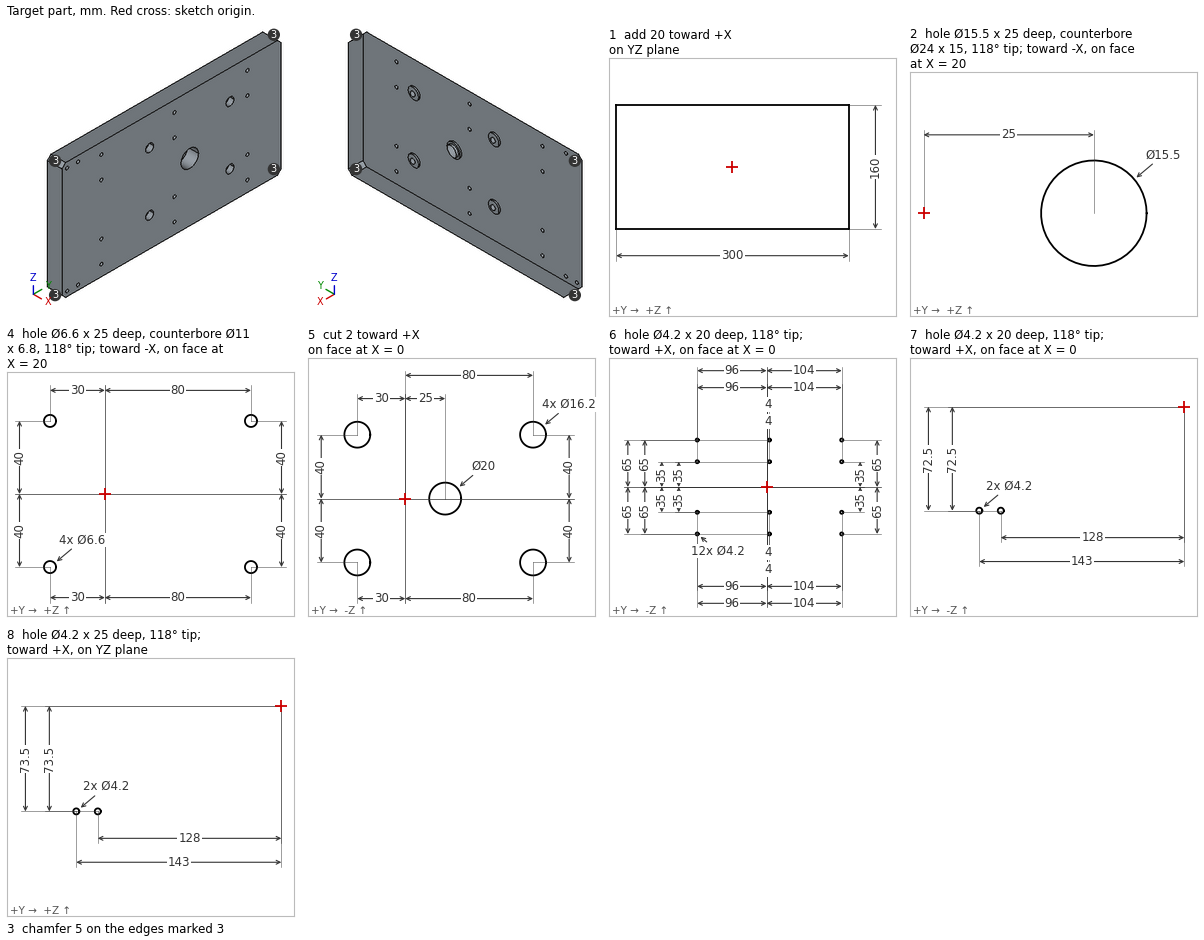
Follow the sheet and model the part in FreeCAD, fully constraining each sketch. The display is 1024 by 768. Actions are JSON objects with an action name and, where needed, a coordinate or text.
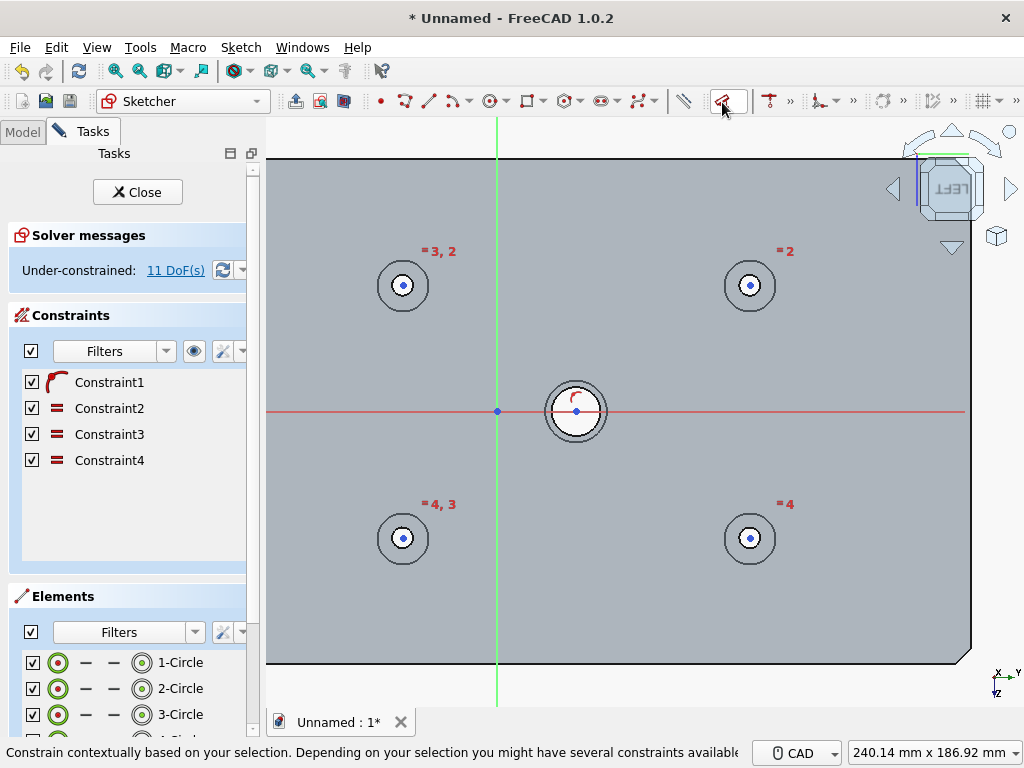
{"action": "left_click", "coordinate": [768, 268]}
{"action": "left_click", "coordinate": [791, 245]}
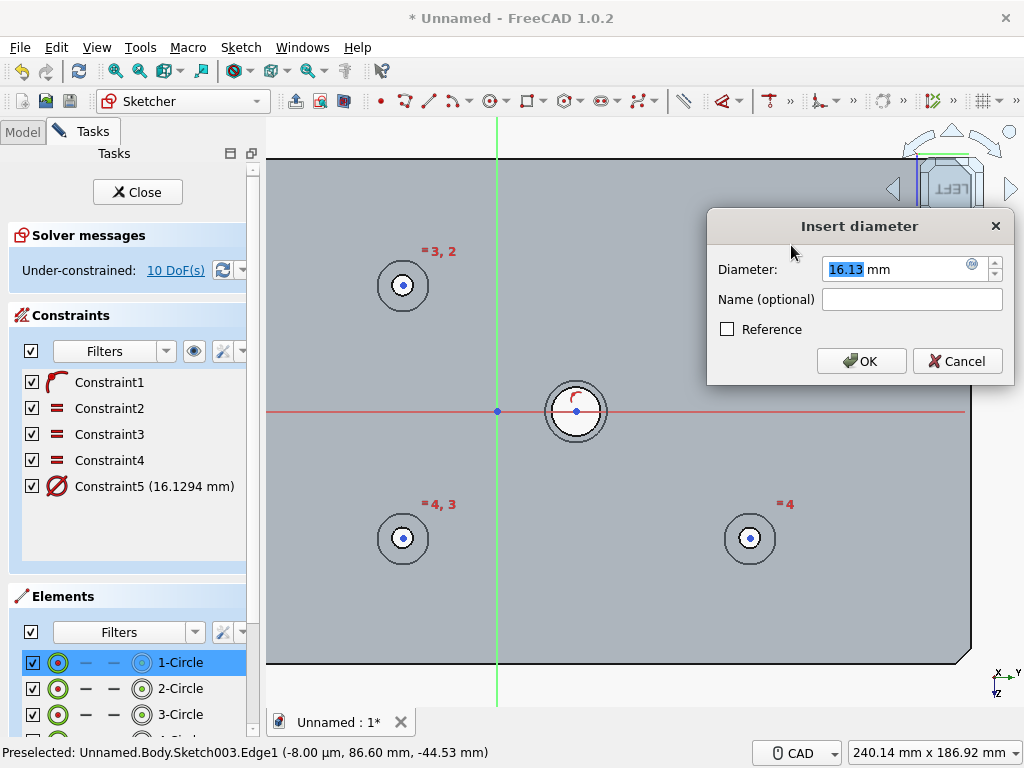
{"action": "type", "text": "16.2"}
{"action": "key", "text": "Return"}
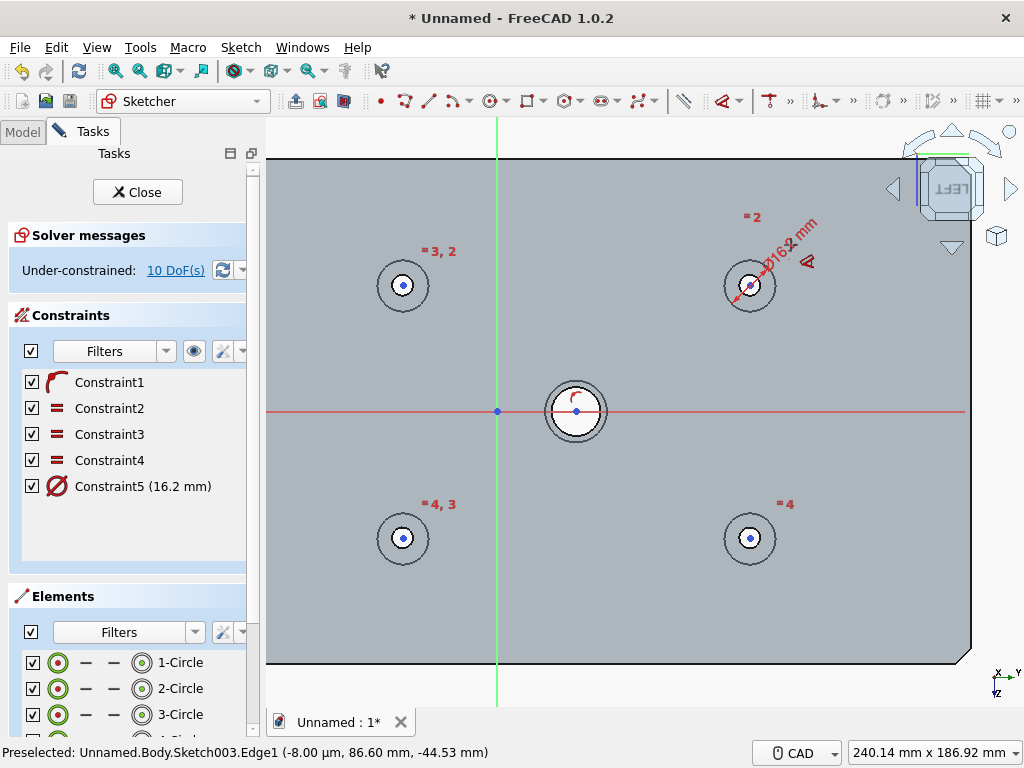
{"action": "left_click", "coordinate": [598, 390]}
{"action": "left_click", "coordinate": [621, 368]}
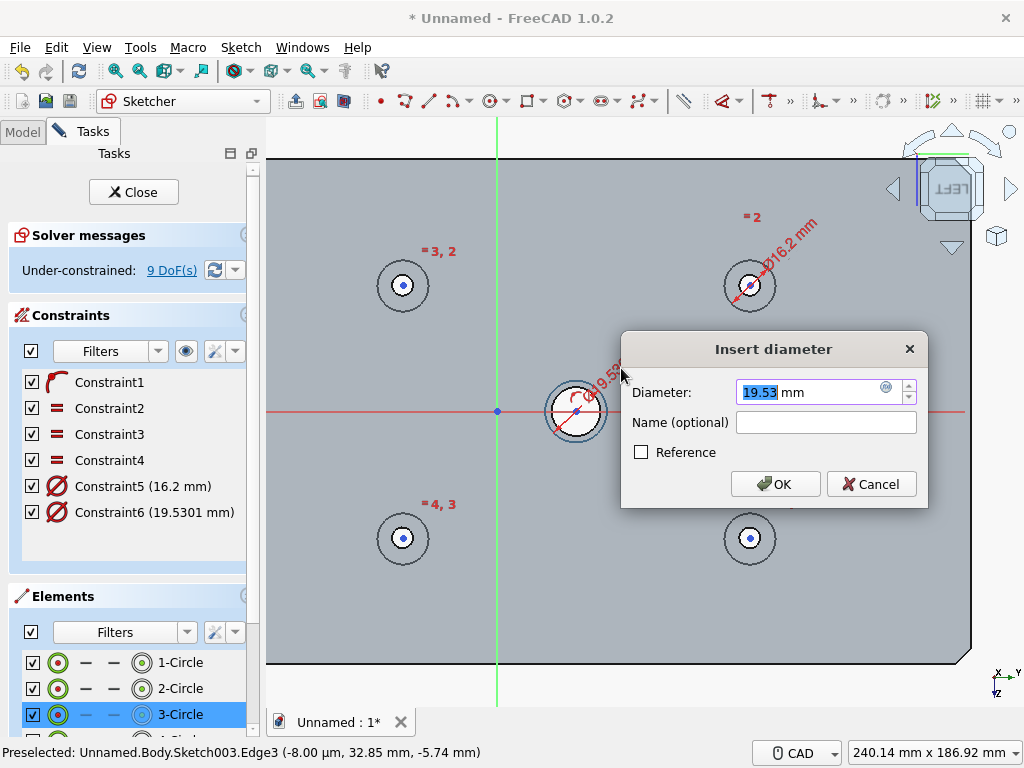
{"action": "type", "text": "20"}
{"action": "key", "text": "Return"}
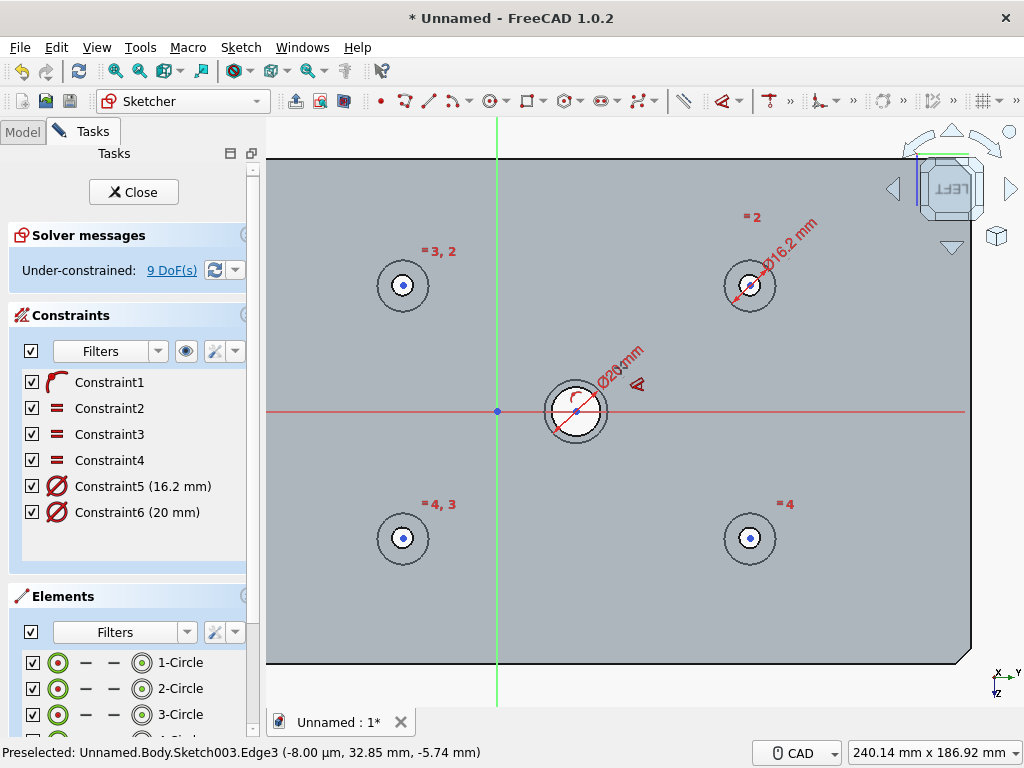
{"action": "left_click", "coordinate": [750, 286]}
{"action": "left_click", "coordinate": [624, 252]}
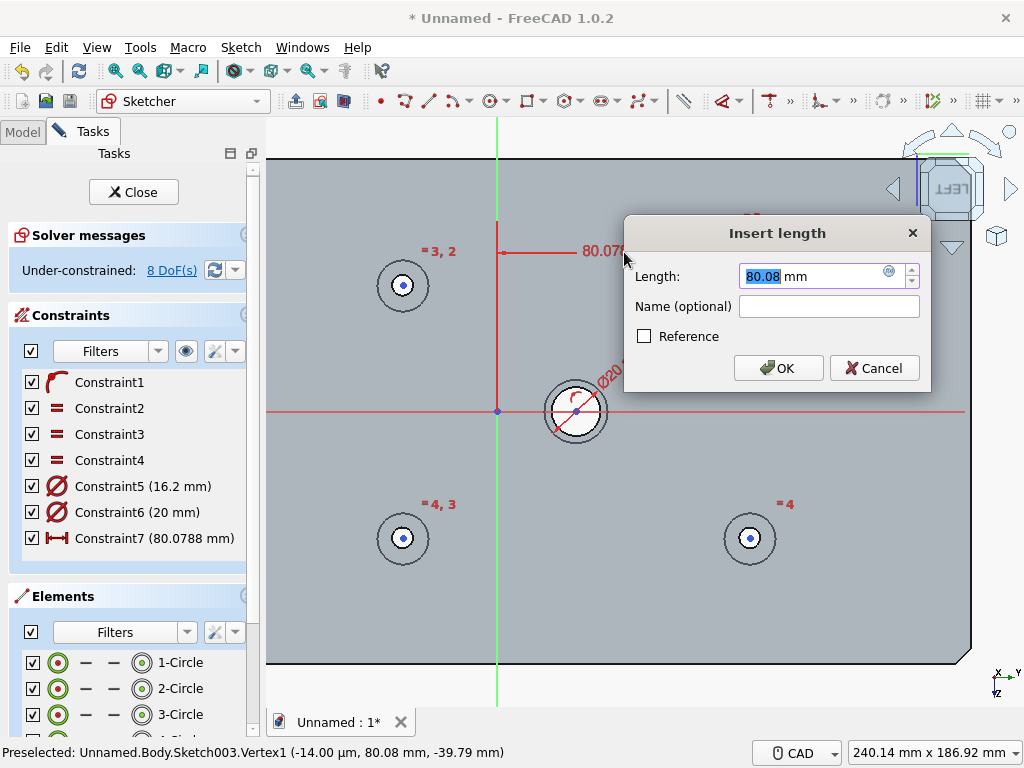
{"action": "type", "text": "80"}
{"action": "key", "text": "Return"}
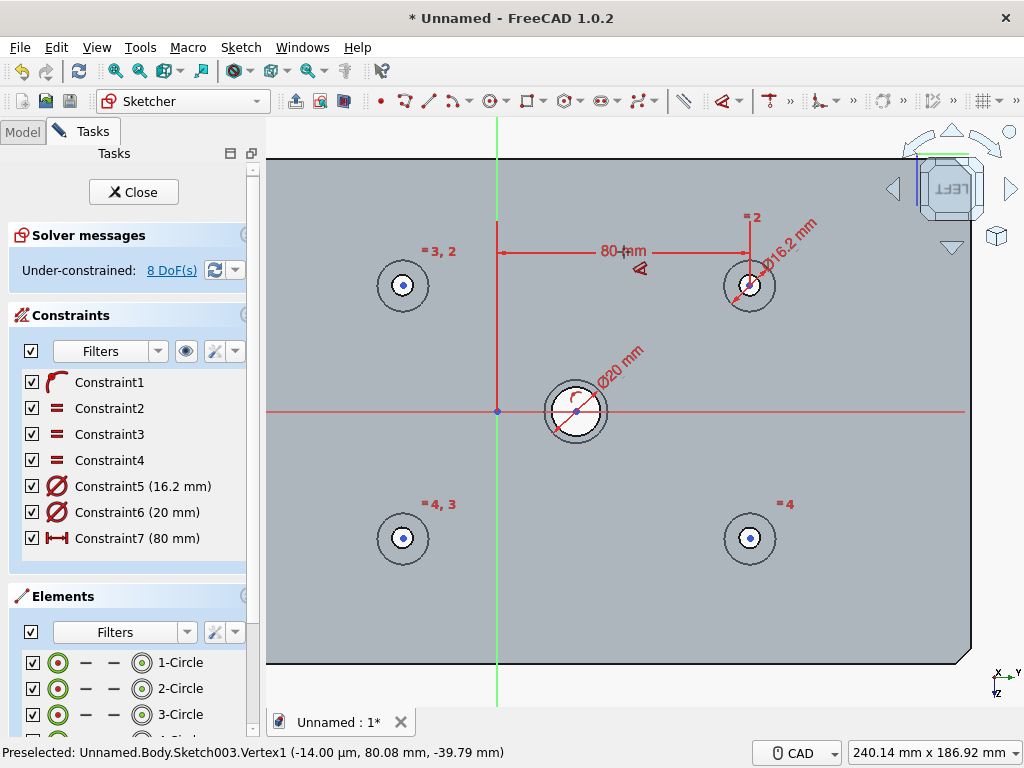
{"action": "left_click", "coordinate": [750, 286]}
{"action": "left_click", "coordinate": [784, 349]}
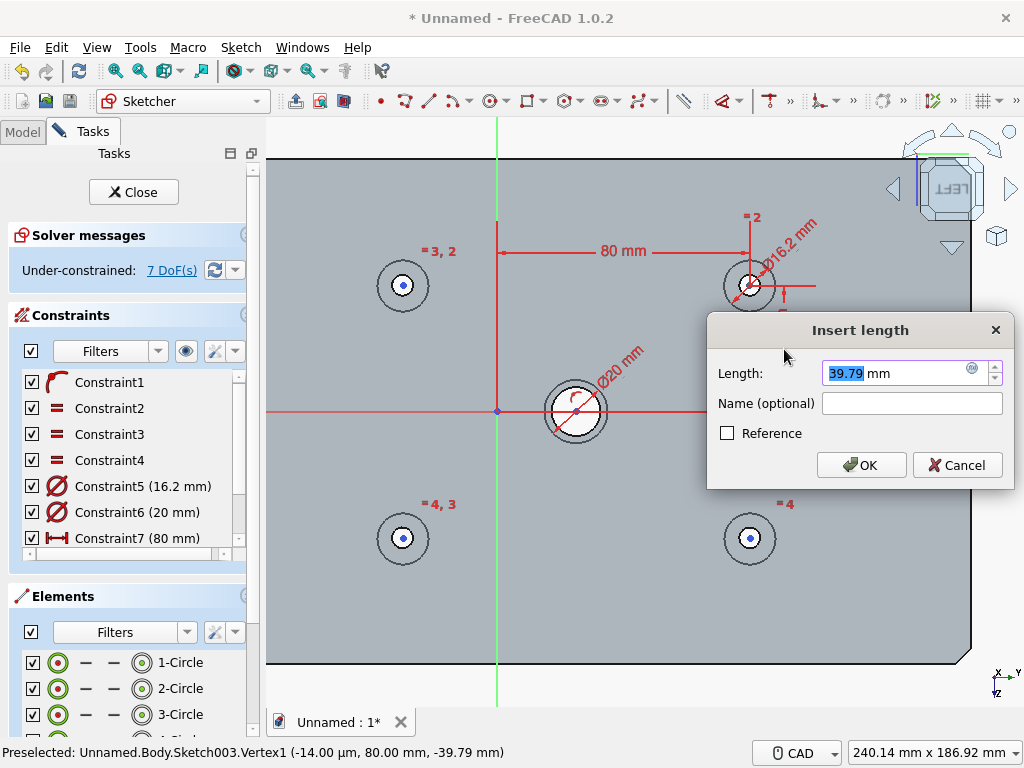
{"action": "type", "text": "40"}
{"action": "key", "text": "Return"}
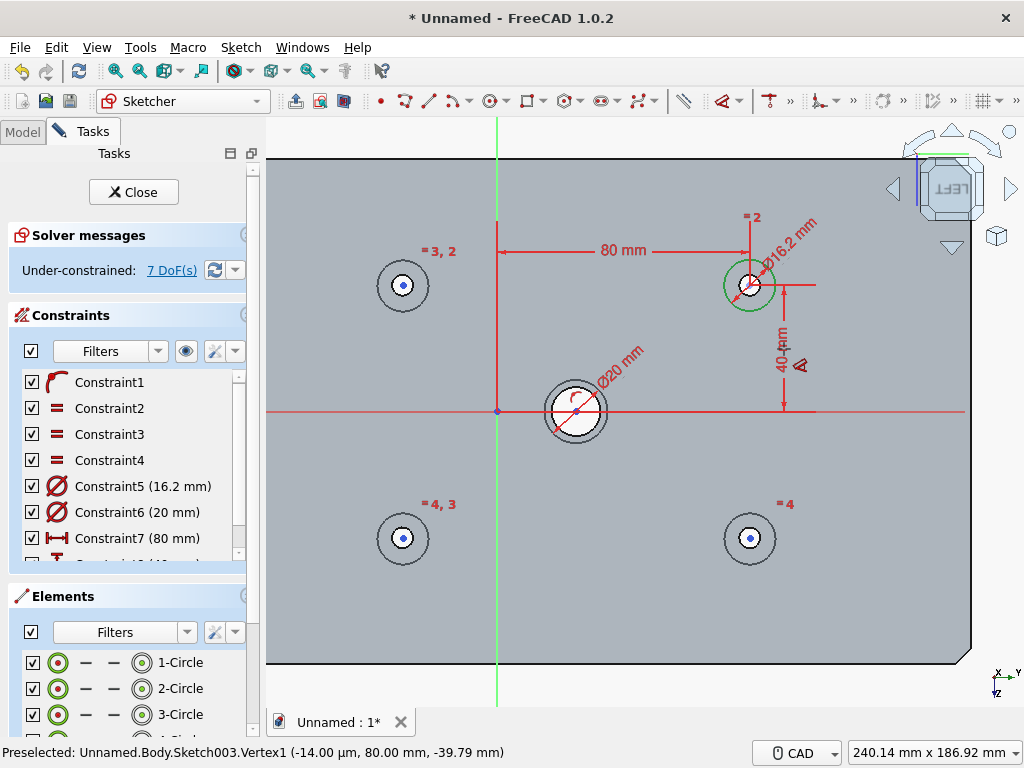
{"action": "left_click", "coordinate": [403, 286]}
{"action": "left_click", "coordinate": [450, 252]}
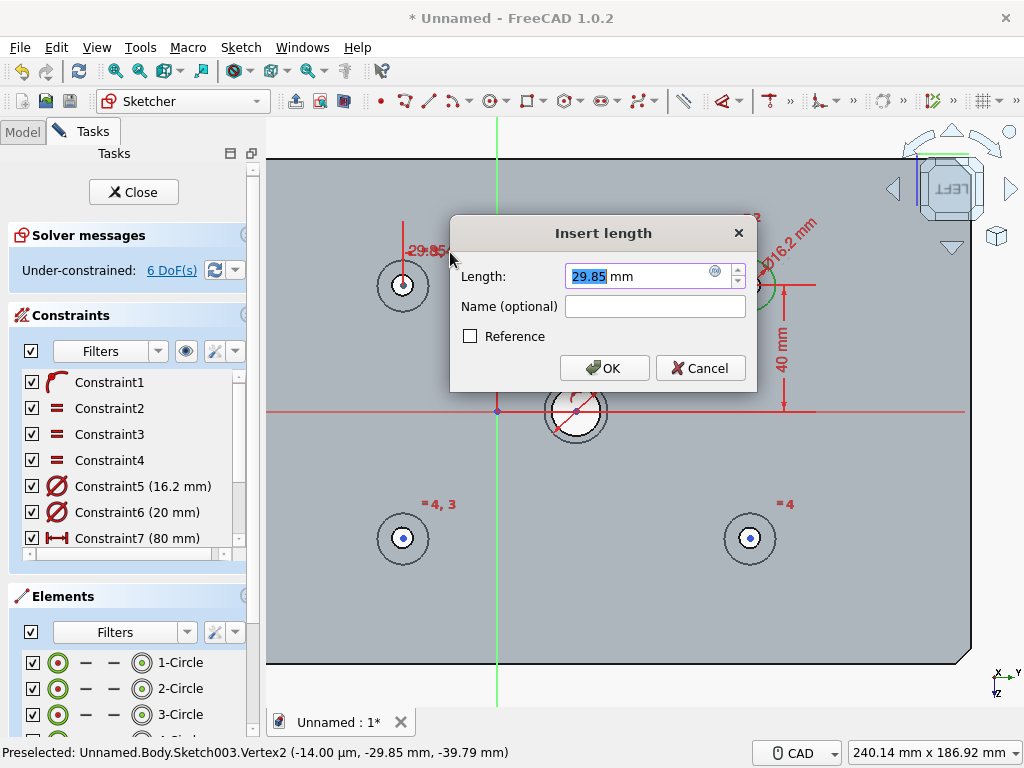
{"action": "type", "text": "30"}
{"action": "key", "text": "Return"}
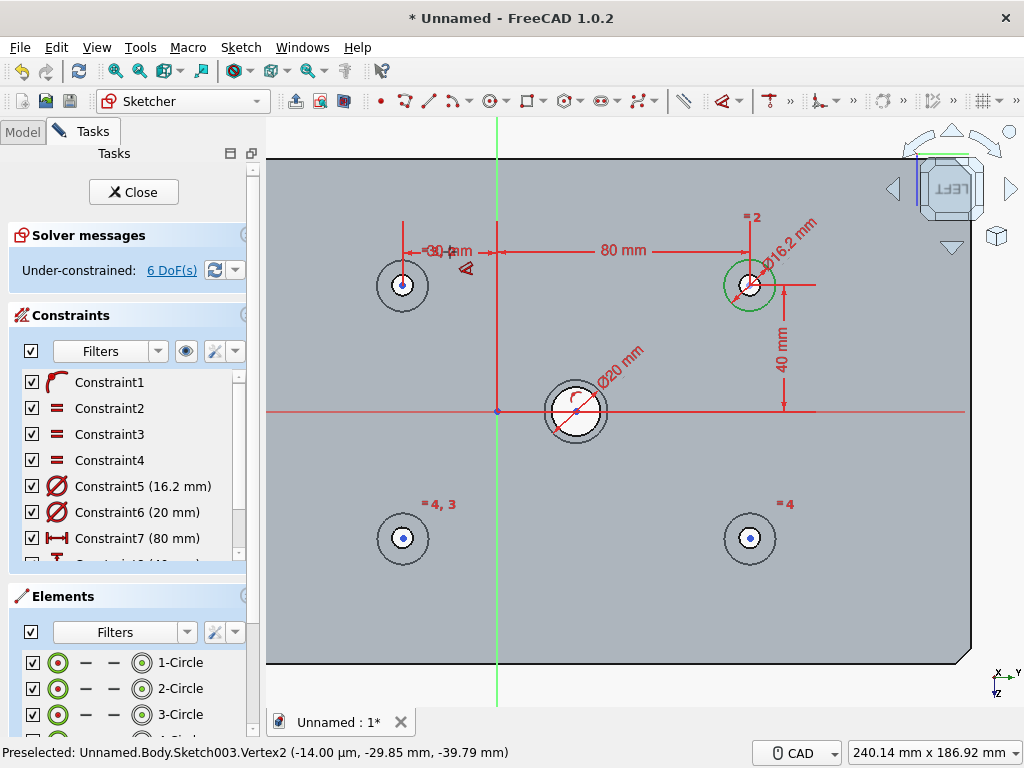
{"action": "left_click", "coordinate": [403, 286]}
{"action": "left_click", "coordinate": [369, 349]}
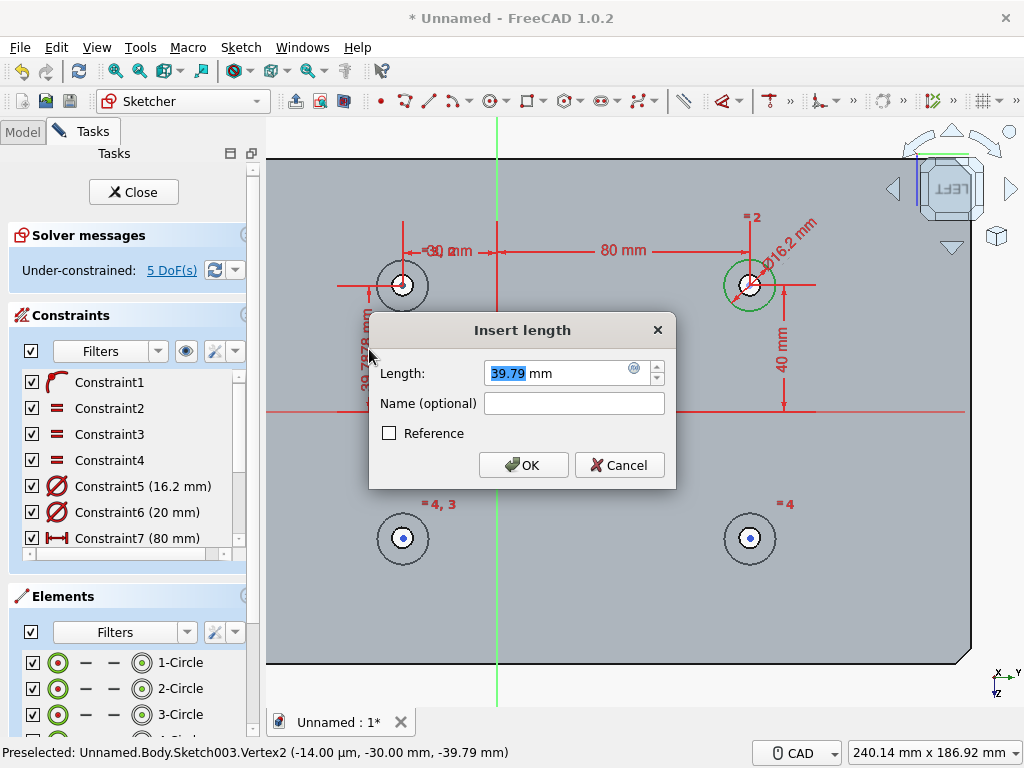
{"action": "type", "text": "40"}
{"action": "key", "text": "Return"}